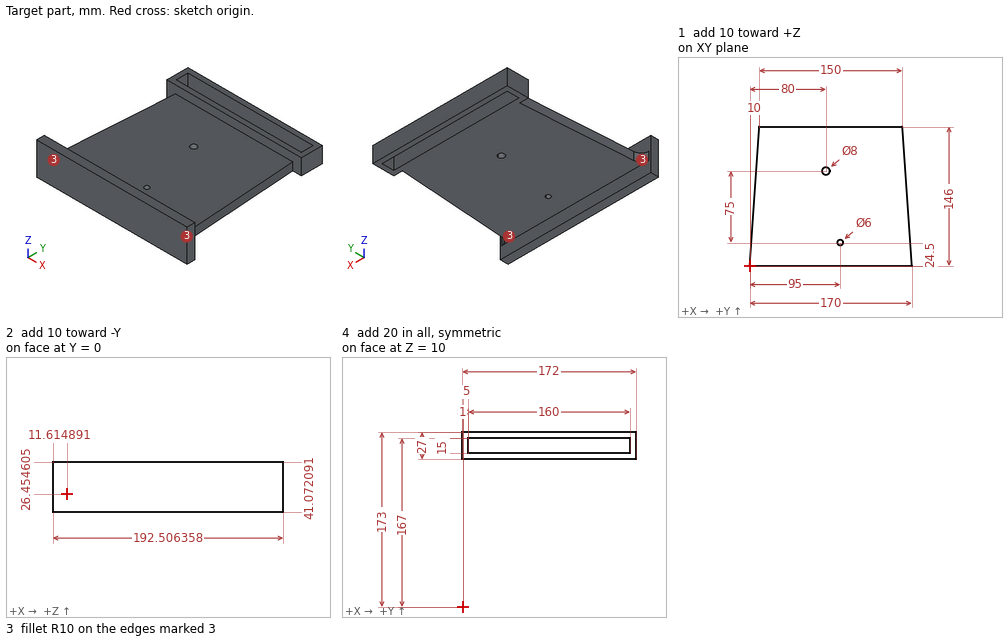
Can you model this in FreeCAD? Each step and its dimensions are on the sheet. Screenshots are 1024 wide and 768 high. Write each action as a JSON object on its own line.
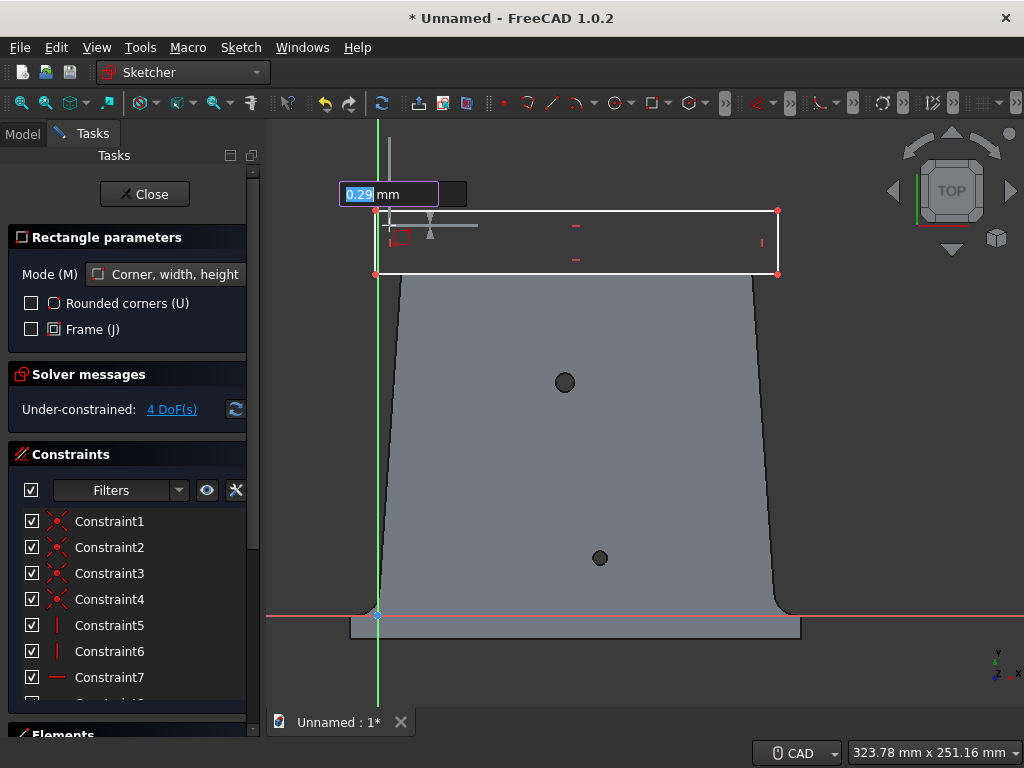
{"action": "left_click", "coordinate": [764, 260]}
{"action": "key", "text": "Escape"}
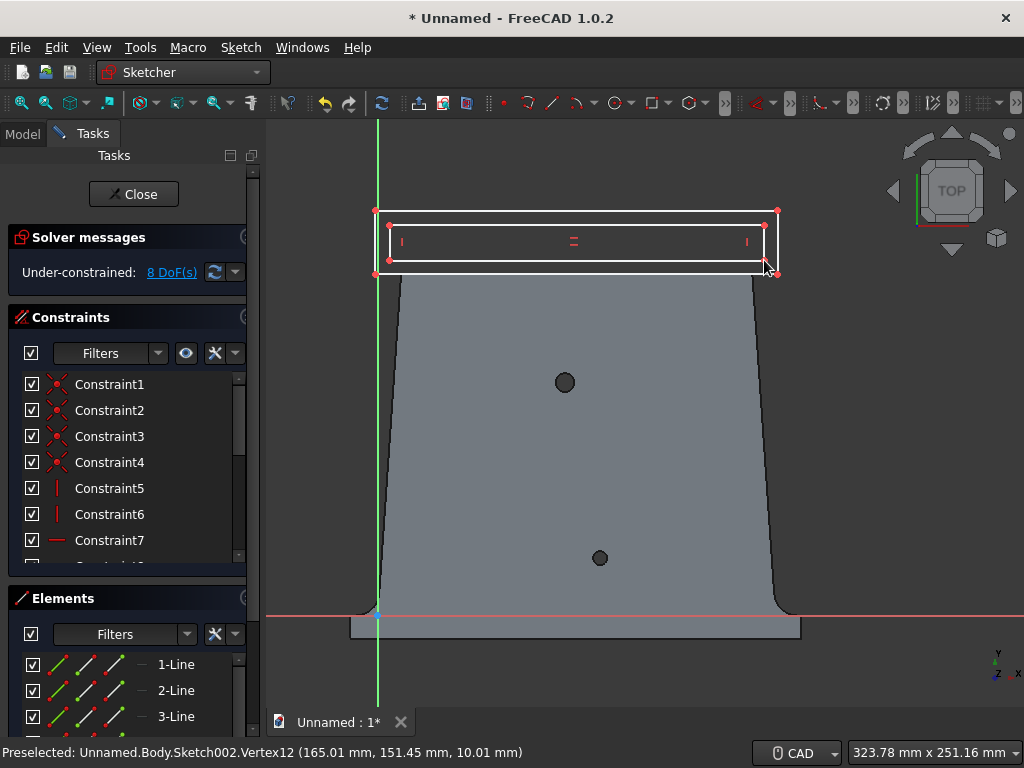
{"action": "left_click", "coordinate": [756, 104]}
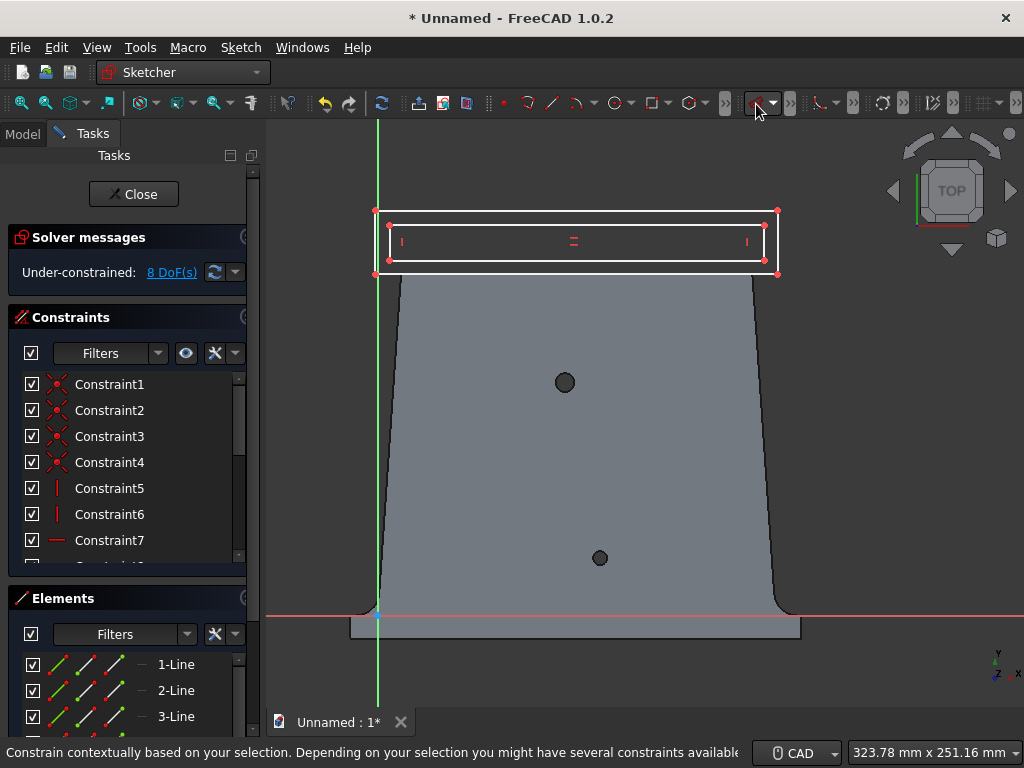
{"action": "left_click", "coordinate": [375, 230]}
{"action": "left_click", "coordinate": [341, 243]}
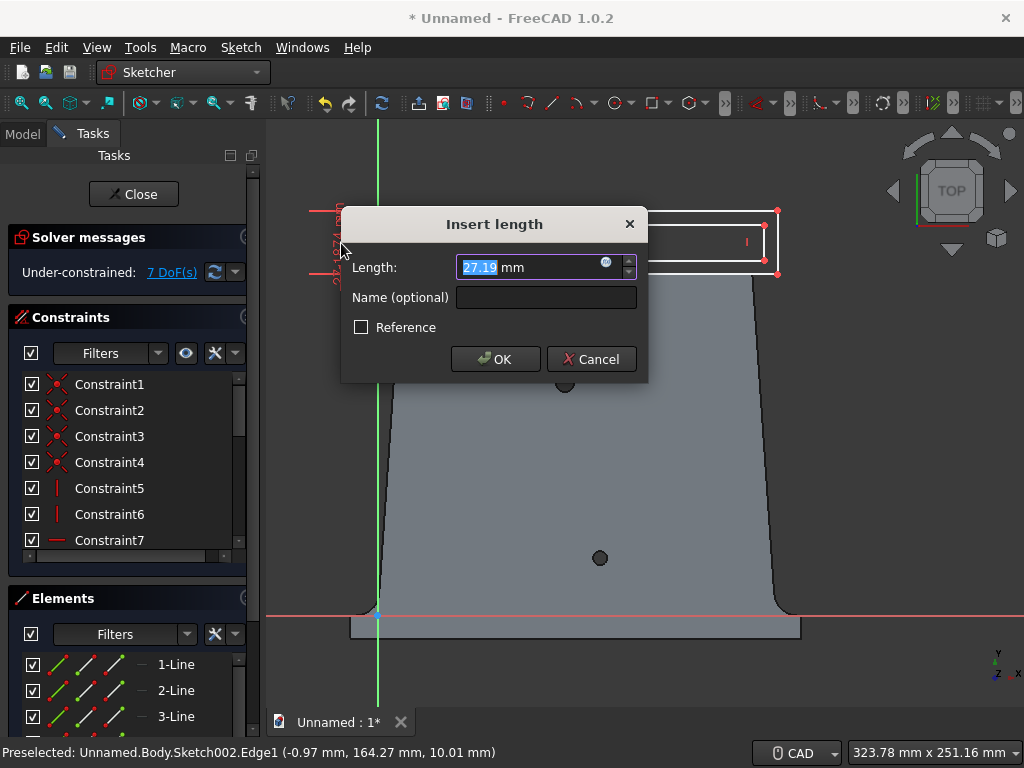
{"action": "type", "text": "27"}
{"action": "key", "text": "Return"}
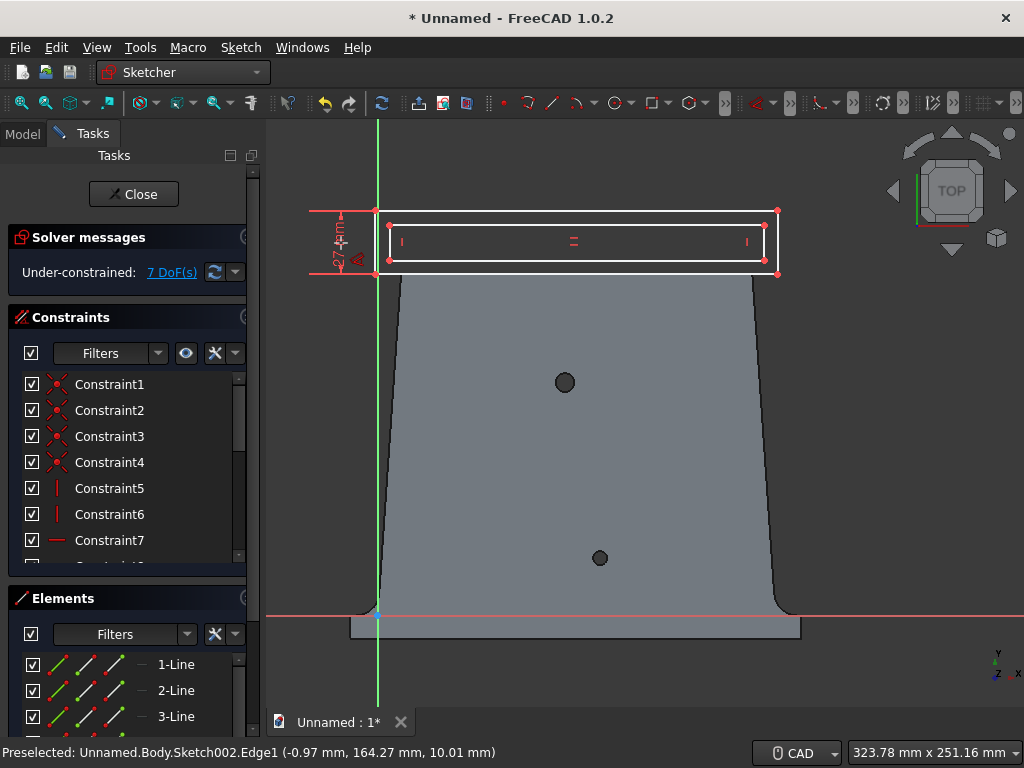
{"action": "scroll", "coordinate": [390, 236], "scroll_direction": "up", "scroll_amount": 2}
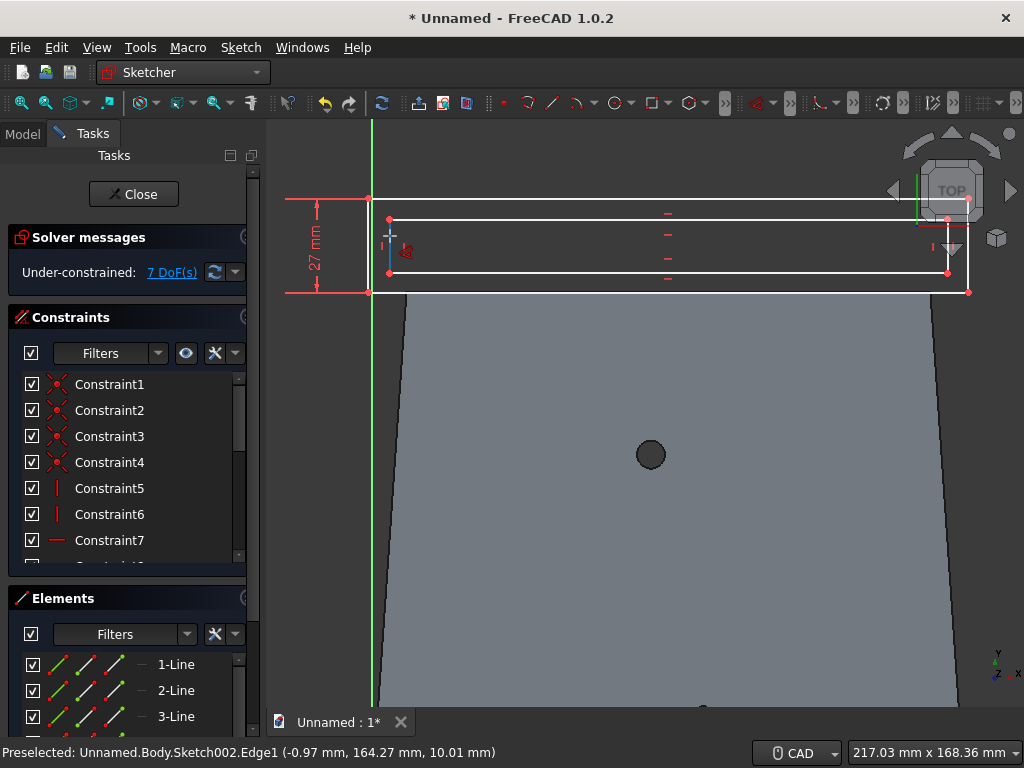
{"action": "left_click", "coordinate": [390, 236]}
{"action": "left_click", "coordinate": [424, 246]}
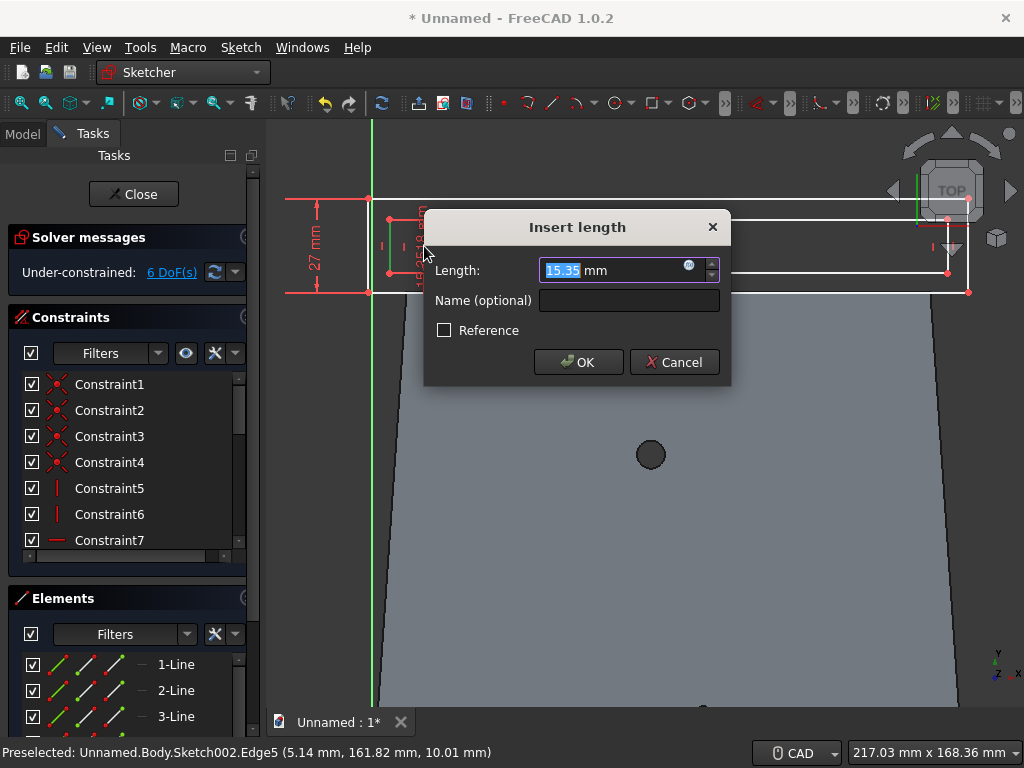
{"action": "type", "text": "15"}
{"action": "key", "text": "Return"}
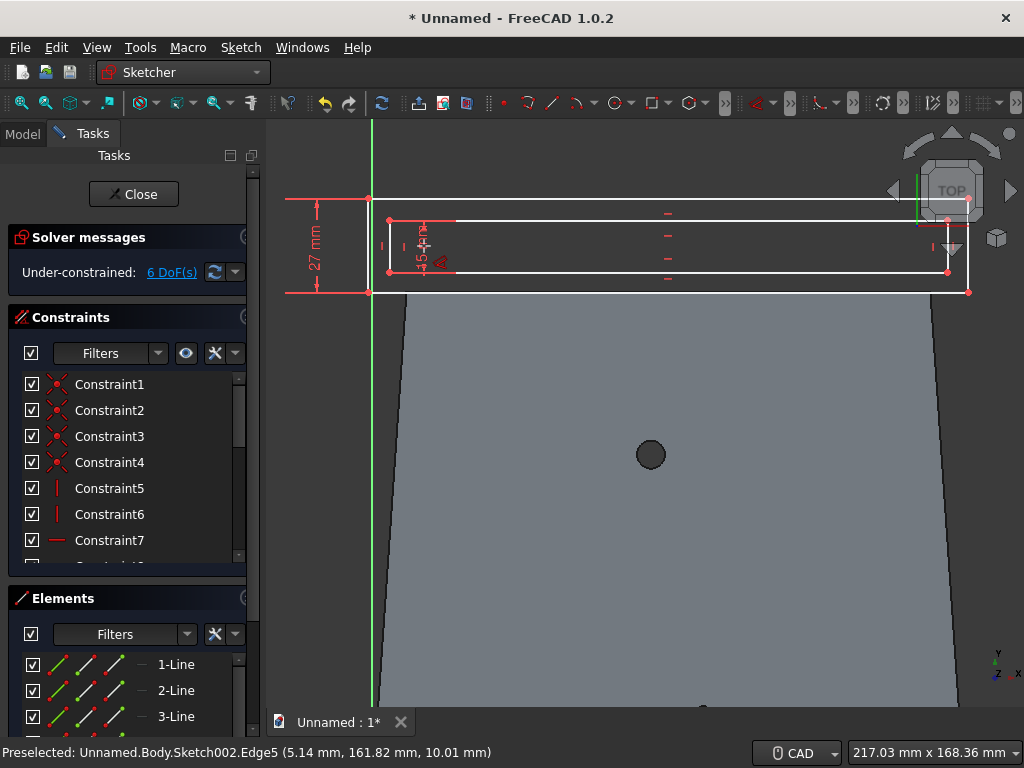
{"action": "scroll", "coordinate": [368, 199], "scroll_direction": "up", "scroll_amount": 13}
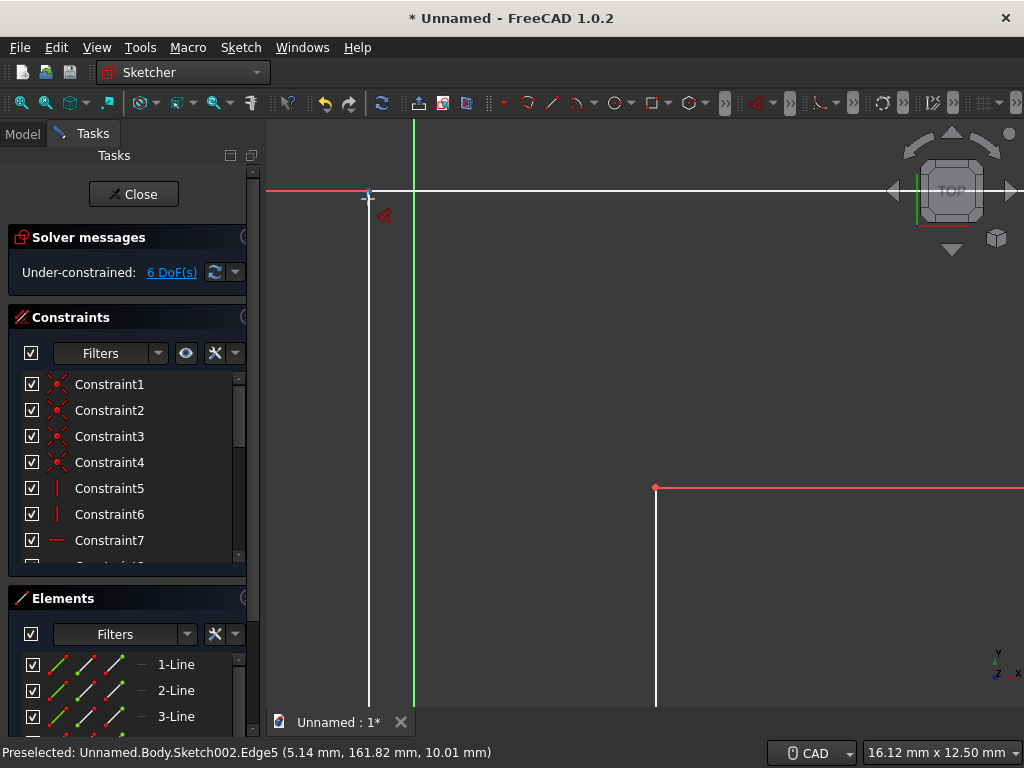
{"action": "left_click", "coordinate": [369, 191]}
{"action": "left_click", "coordinate": [391, 157]}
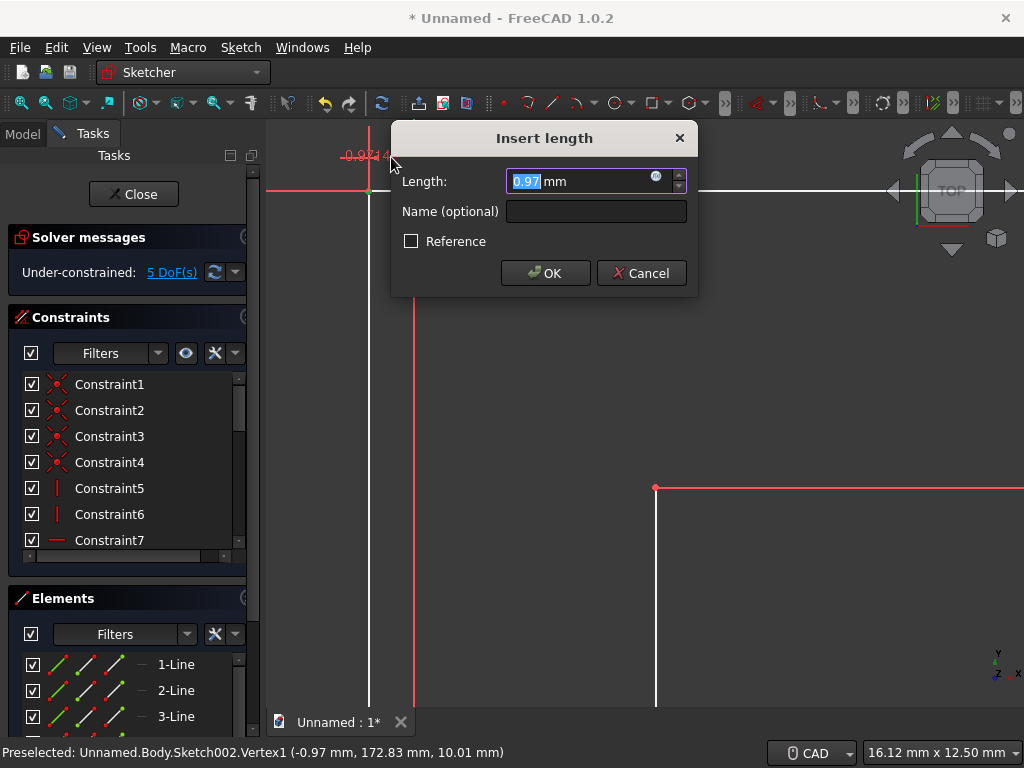
{"action": "type", "text": "1"}
{"action": "key", "text": "Return"}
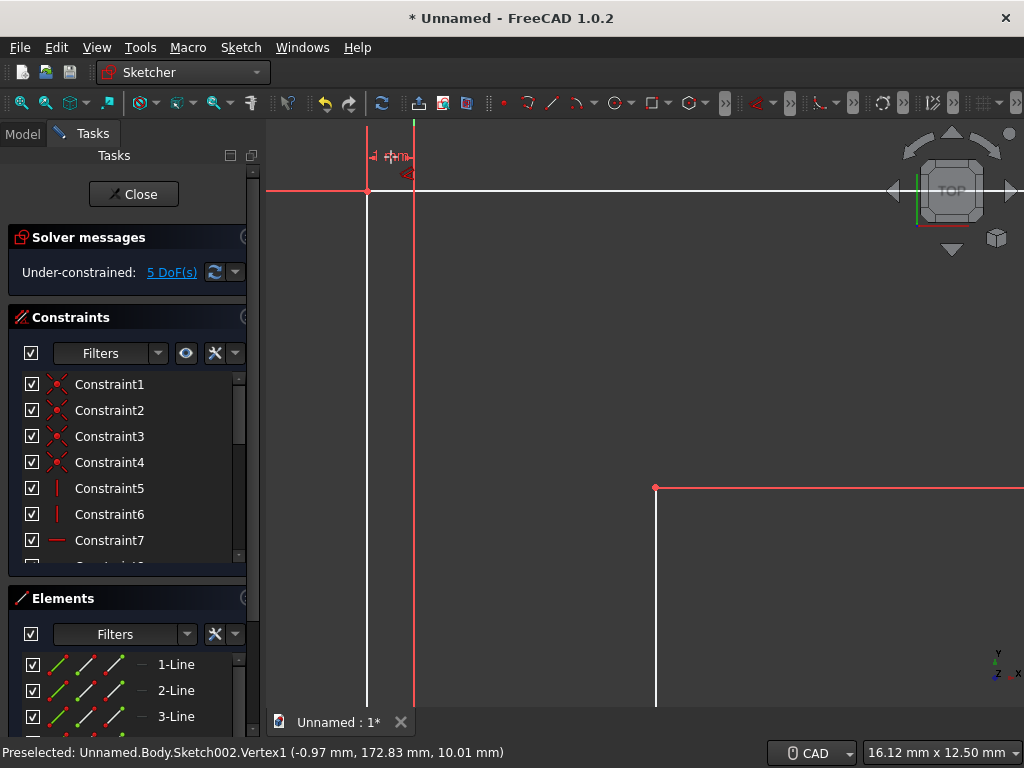
{"action": "scroll", "coordinate": [376, 212], "scroll_direction": "down", "scroll_amount": 15}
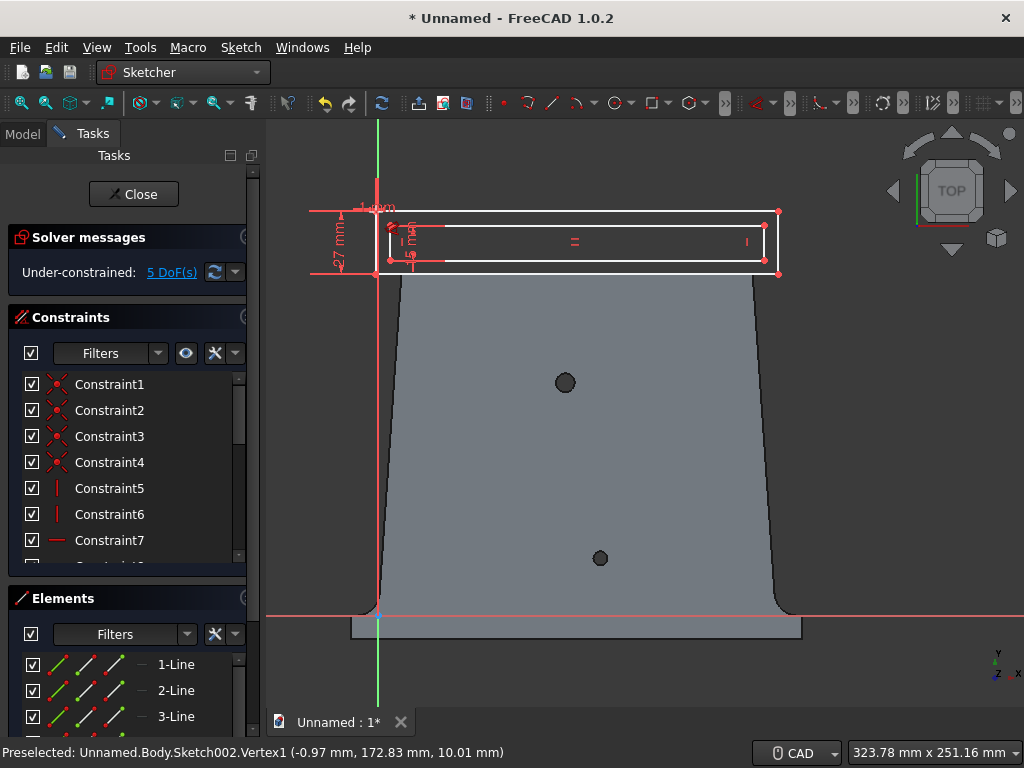
{"action": "scroll", "coordinate": [390, 226], "scroll_direction": "up", "scroll_amount": 7}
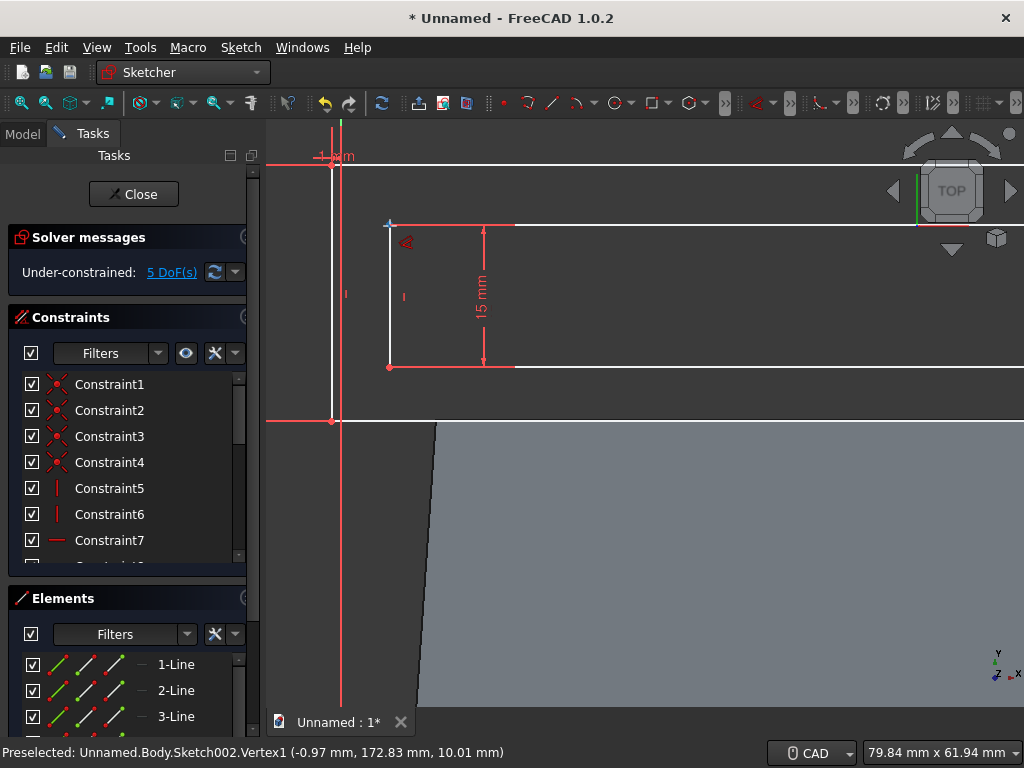
{"action": "left_click", "coordinate": [390, 225]}
{"action": "left_click", "coordinate": [365, 191]}